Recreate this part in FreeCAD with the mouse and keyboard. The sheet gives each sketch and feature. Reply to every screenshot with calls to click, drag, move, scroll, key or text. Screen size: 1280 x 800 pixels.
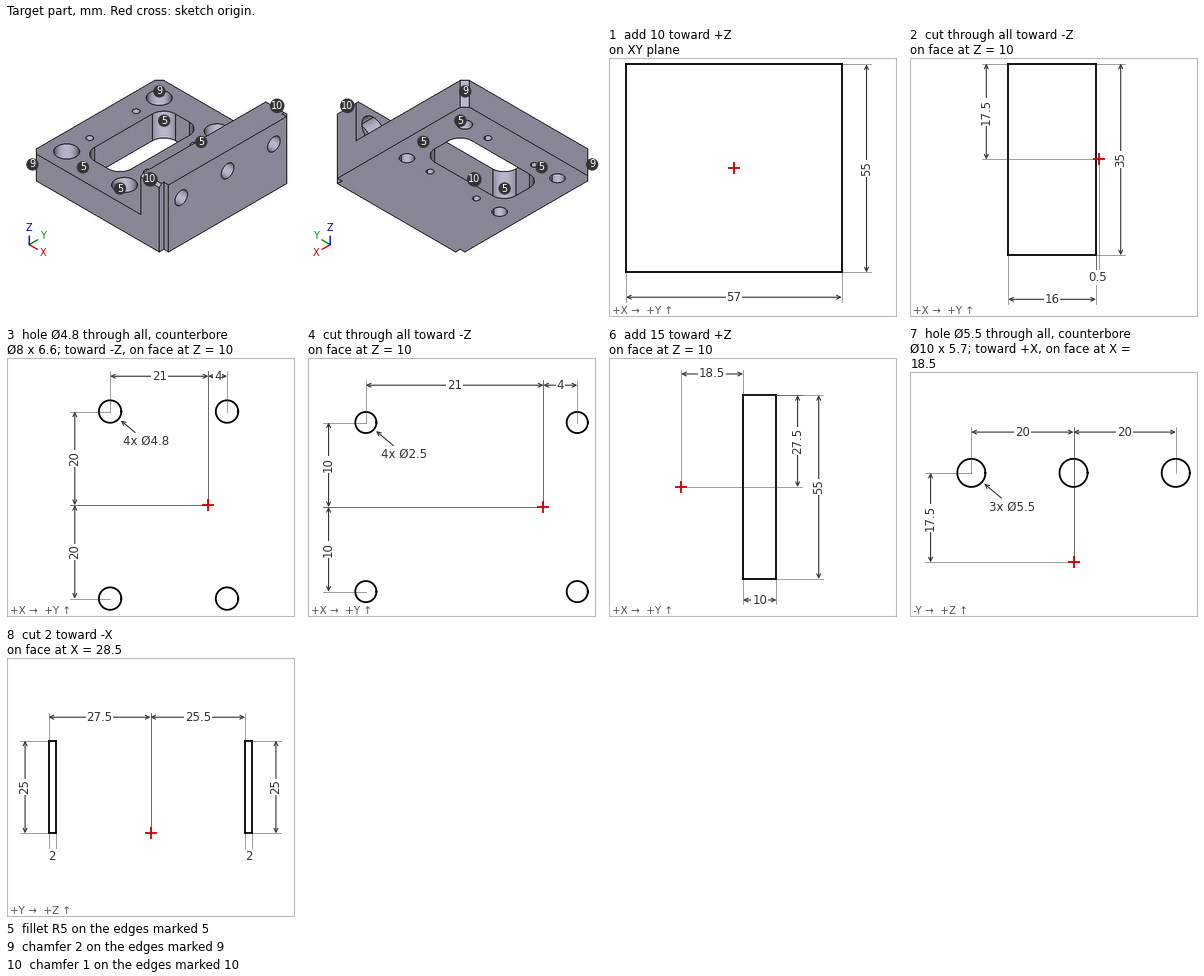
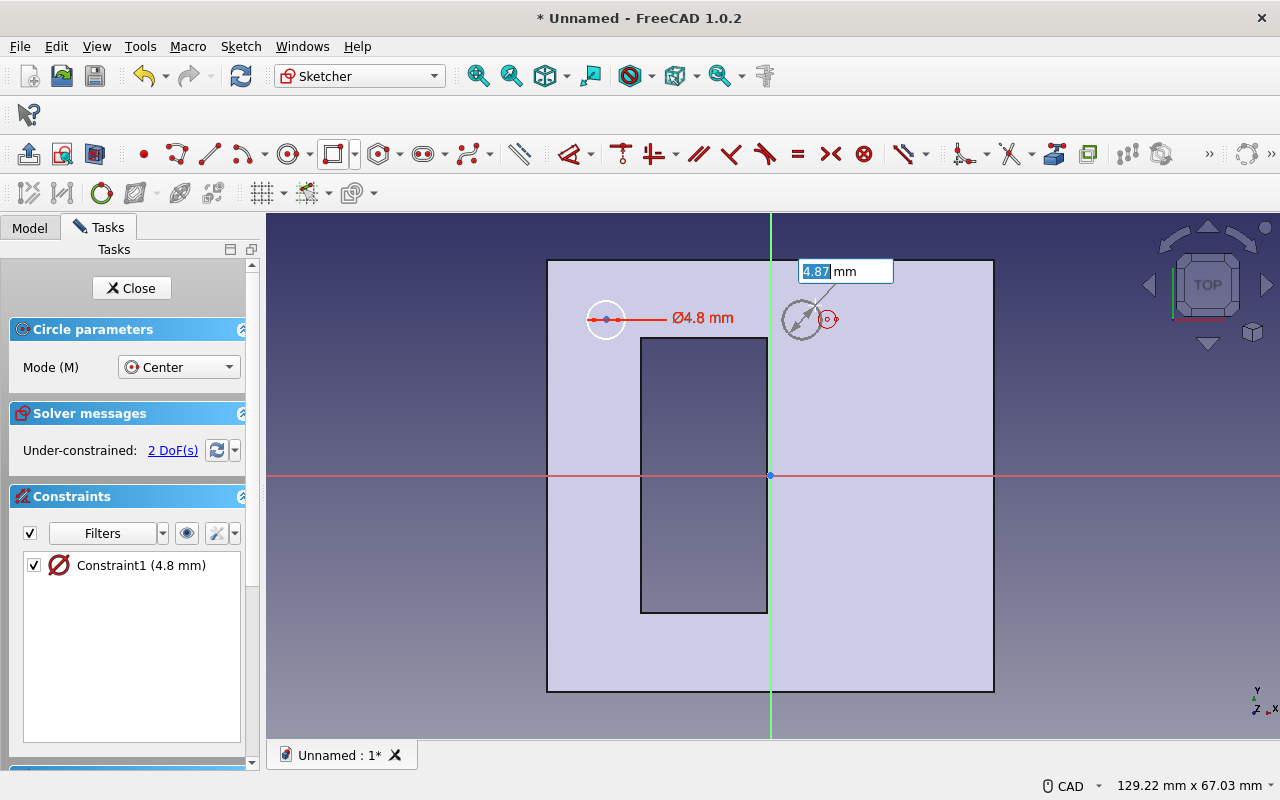
text(4.8)
key(Return)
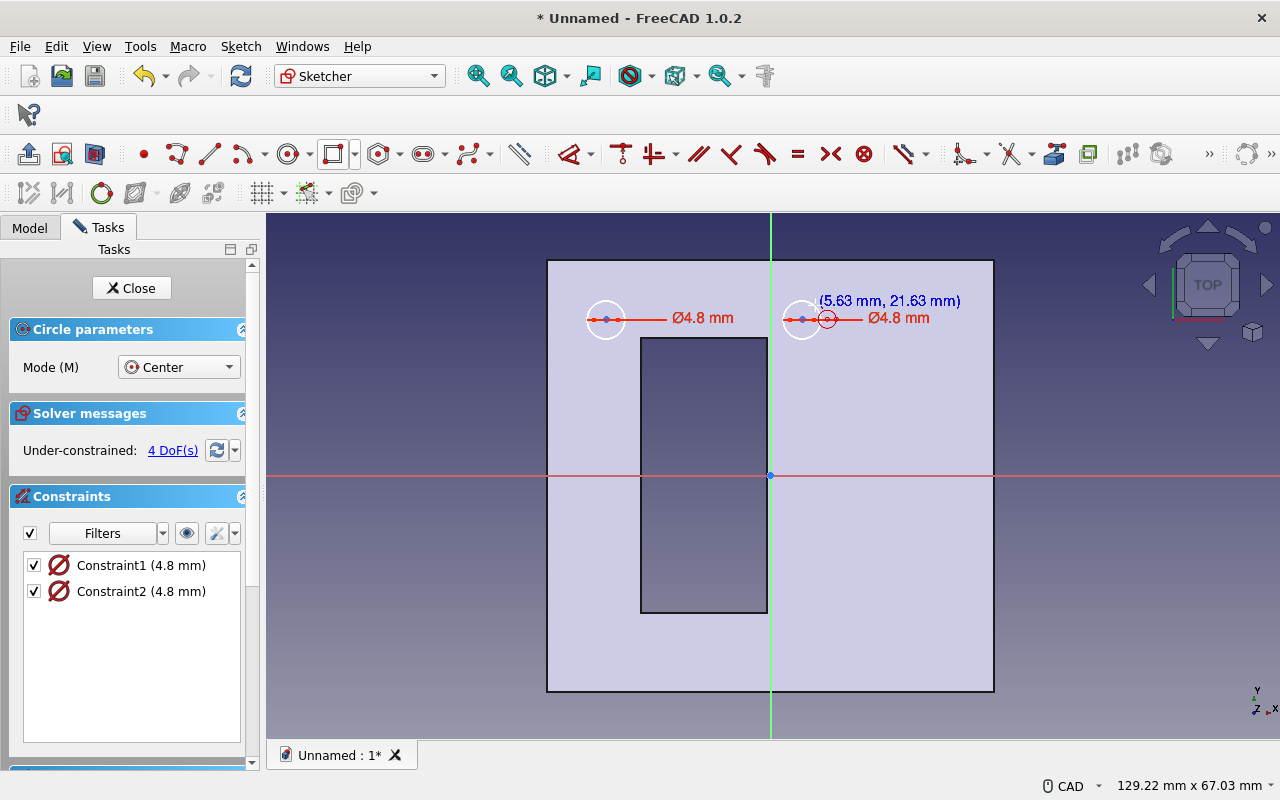
click(606, 633)
move(619, 619)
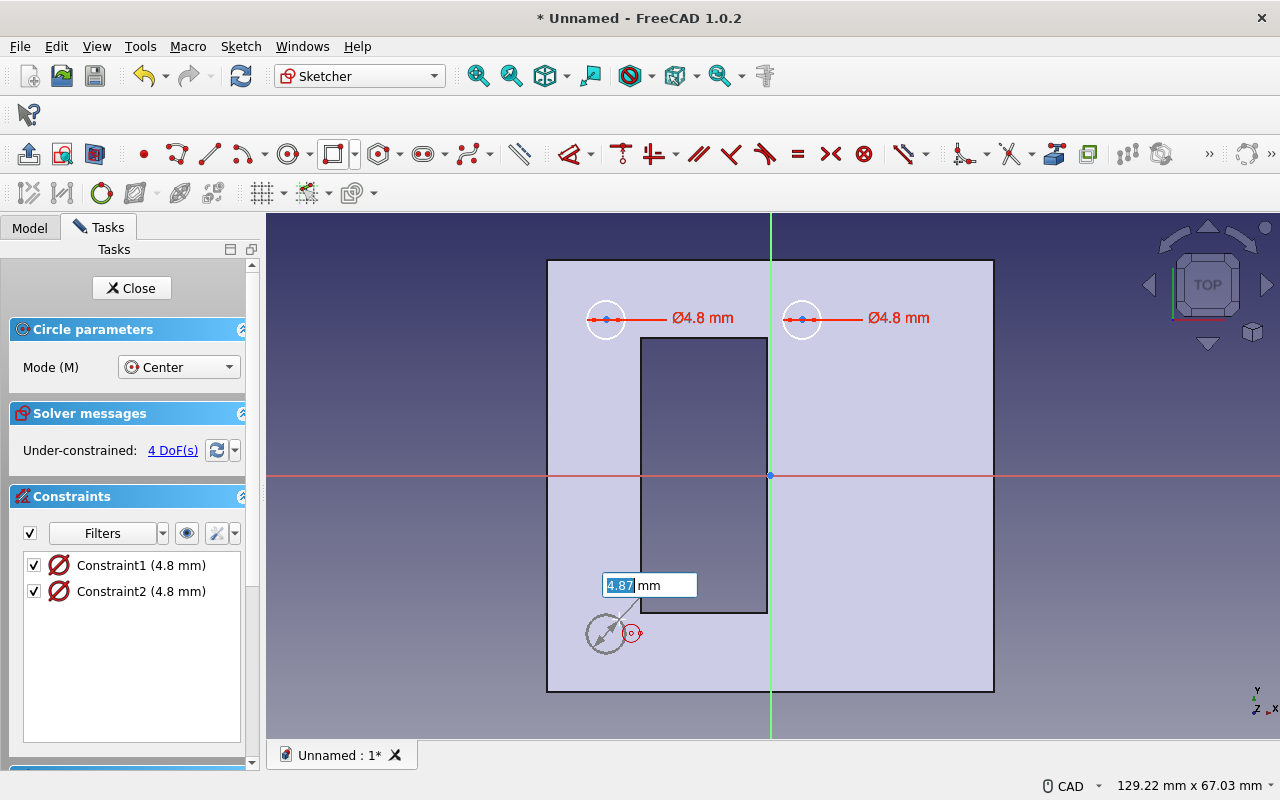
text(4.8)
key(Return)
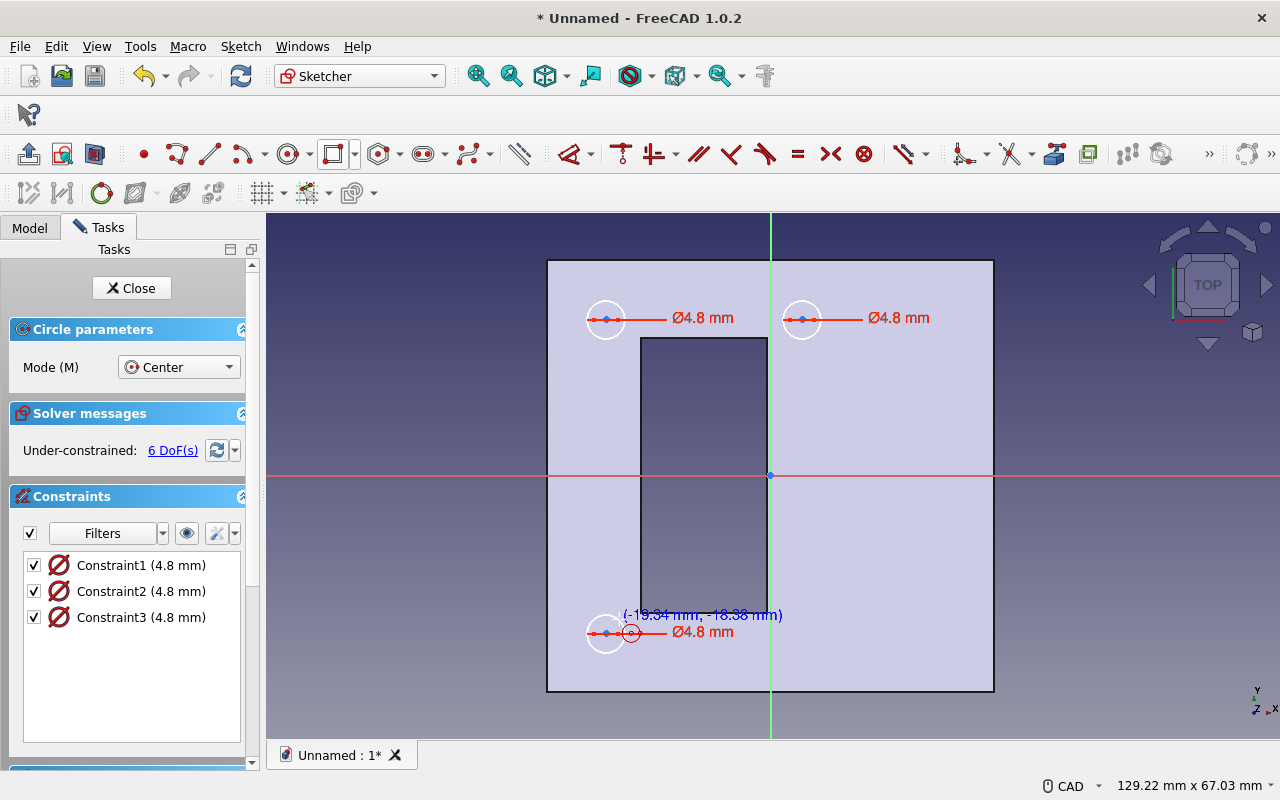
click(802, 633)
move(815, 619)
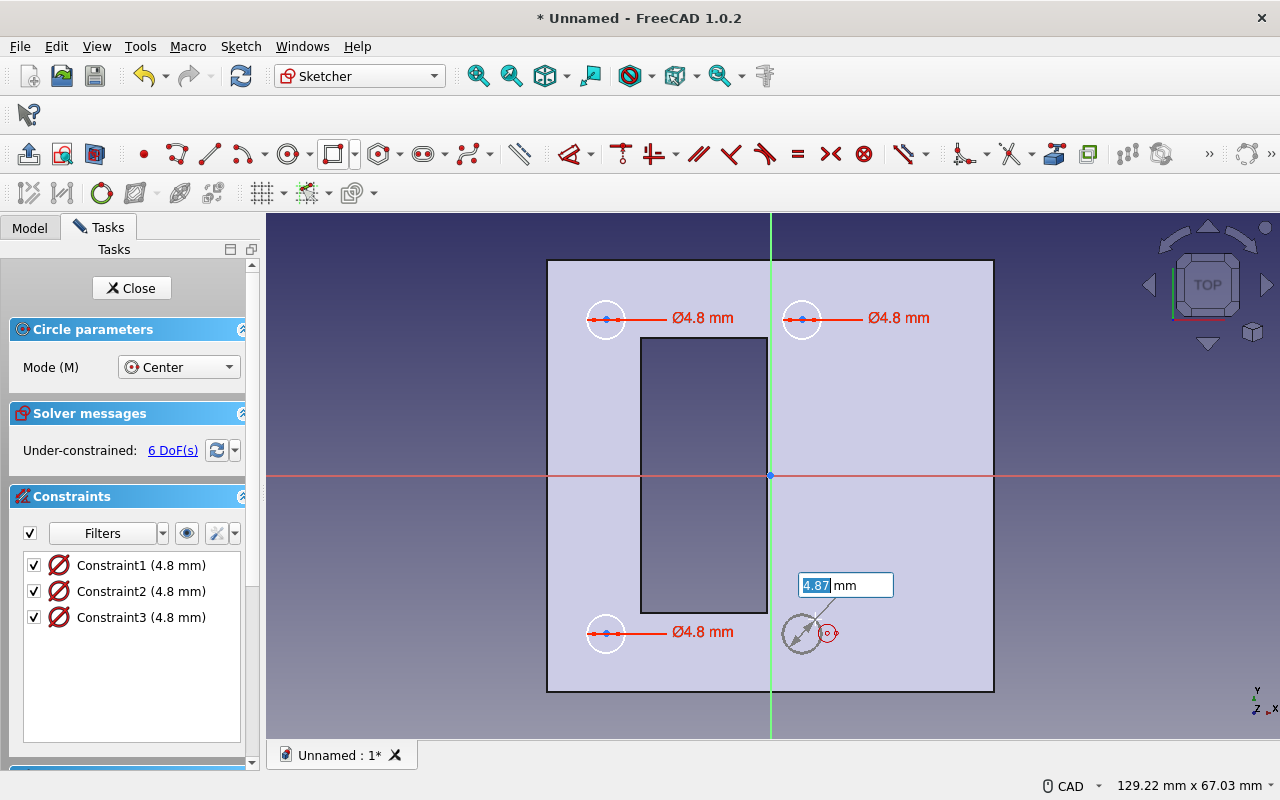
text(4.8)
key(Return)
key(Escape)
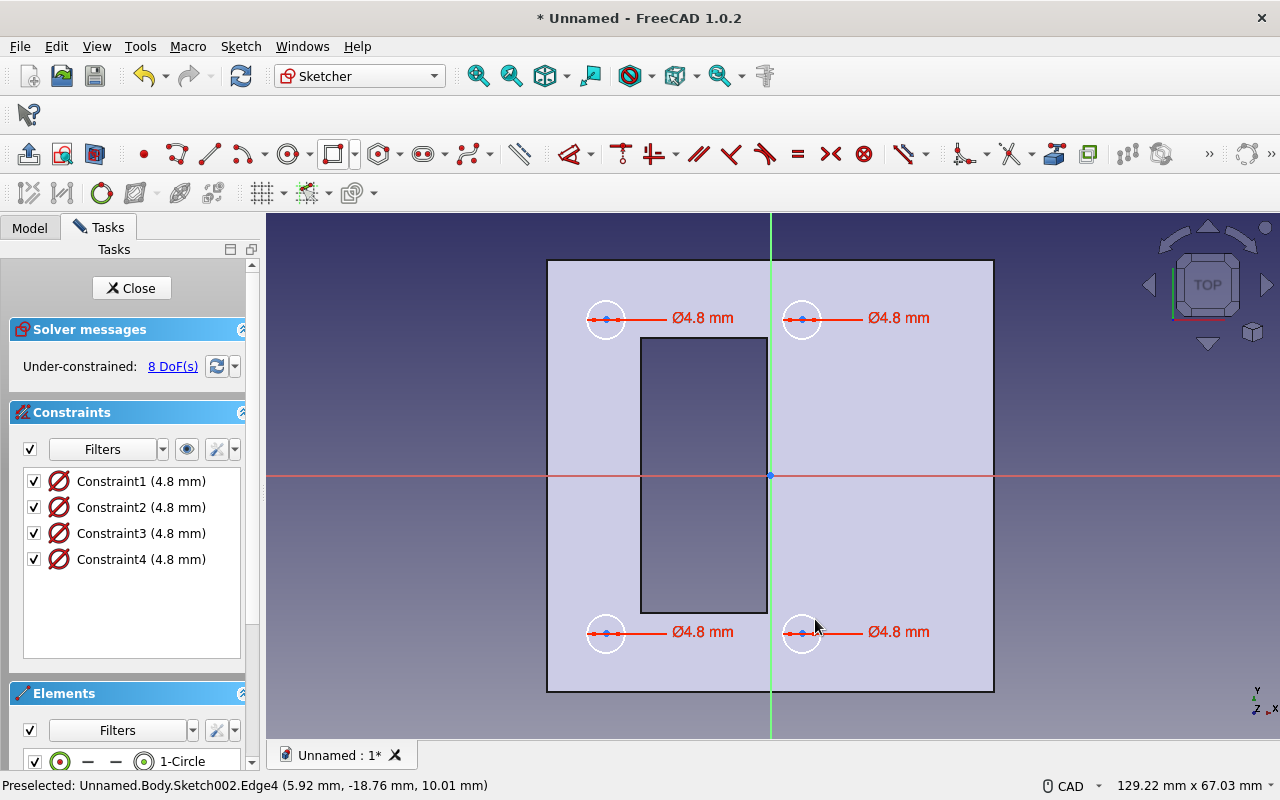
click(606, 320)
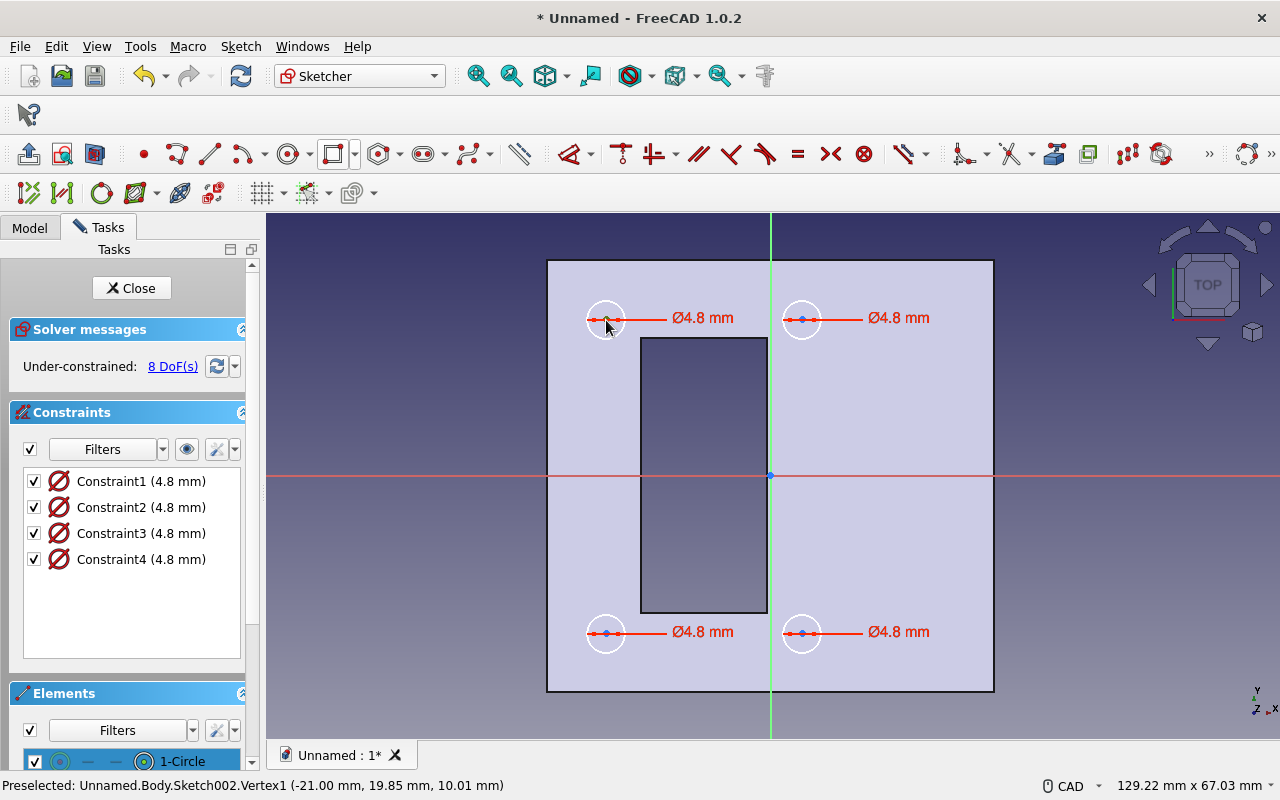
click(802, 320)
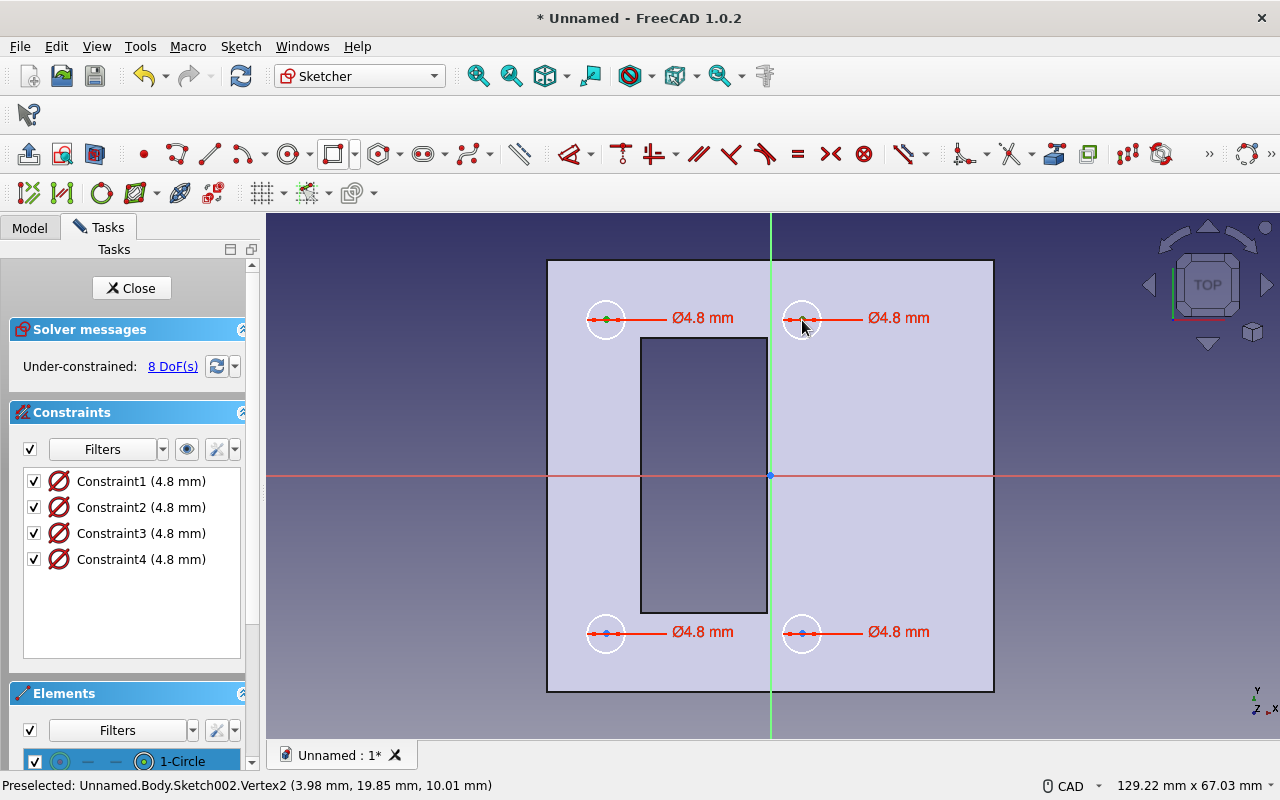
click(676, 154)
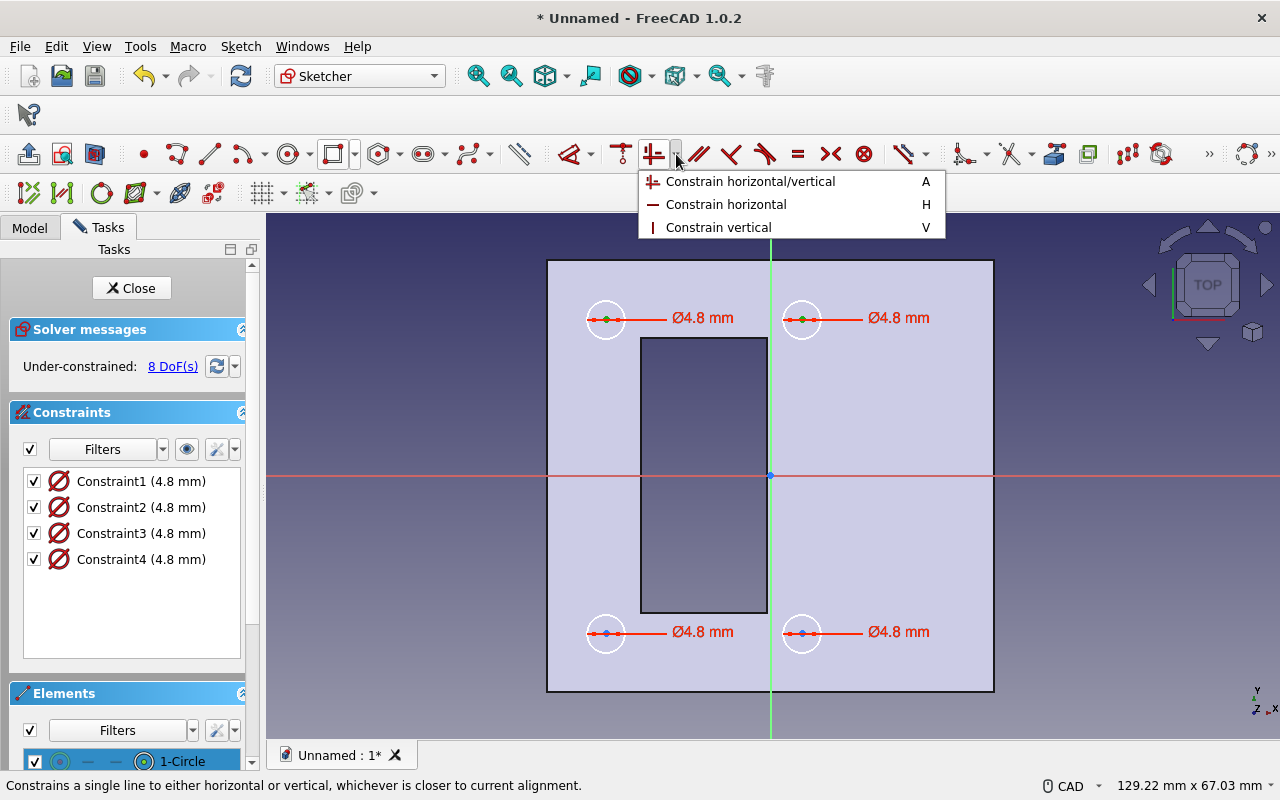
click(792, 204)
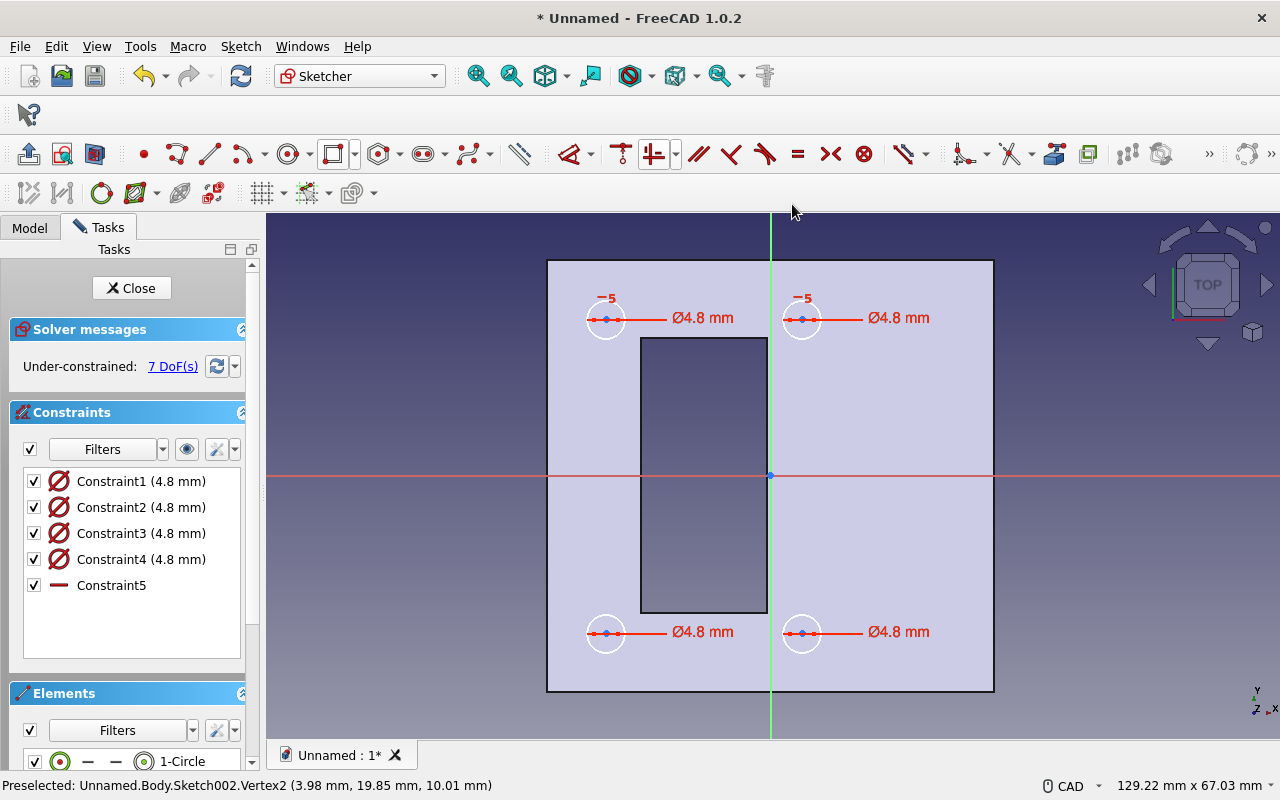
click(606, 320)